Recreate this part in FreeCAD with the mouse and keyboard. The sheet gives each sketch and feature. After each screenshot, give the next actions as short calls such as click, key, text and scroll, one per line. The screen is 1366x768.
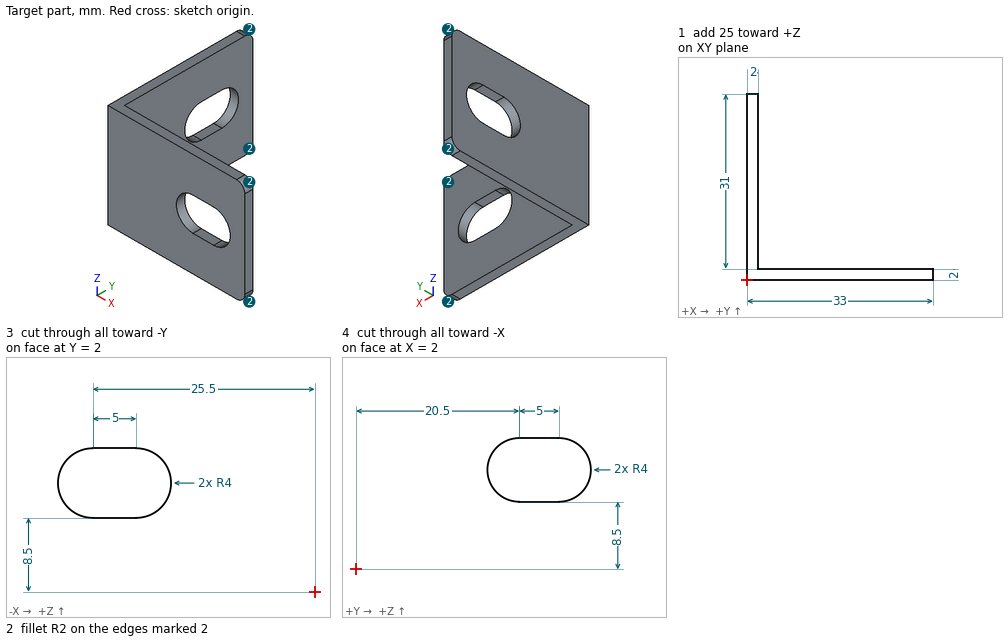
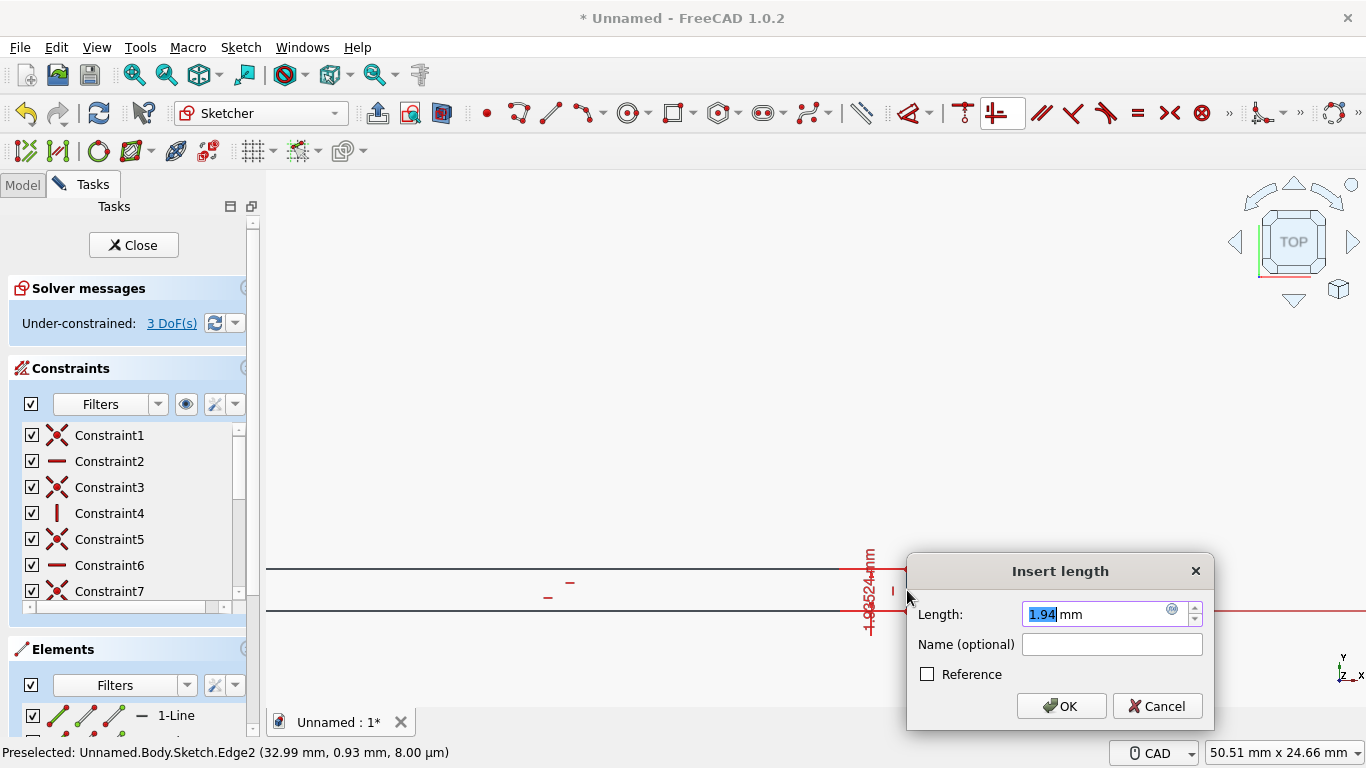
text(2)
key(Return)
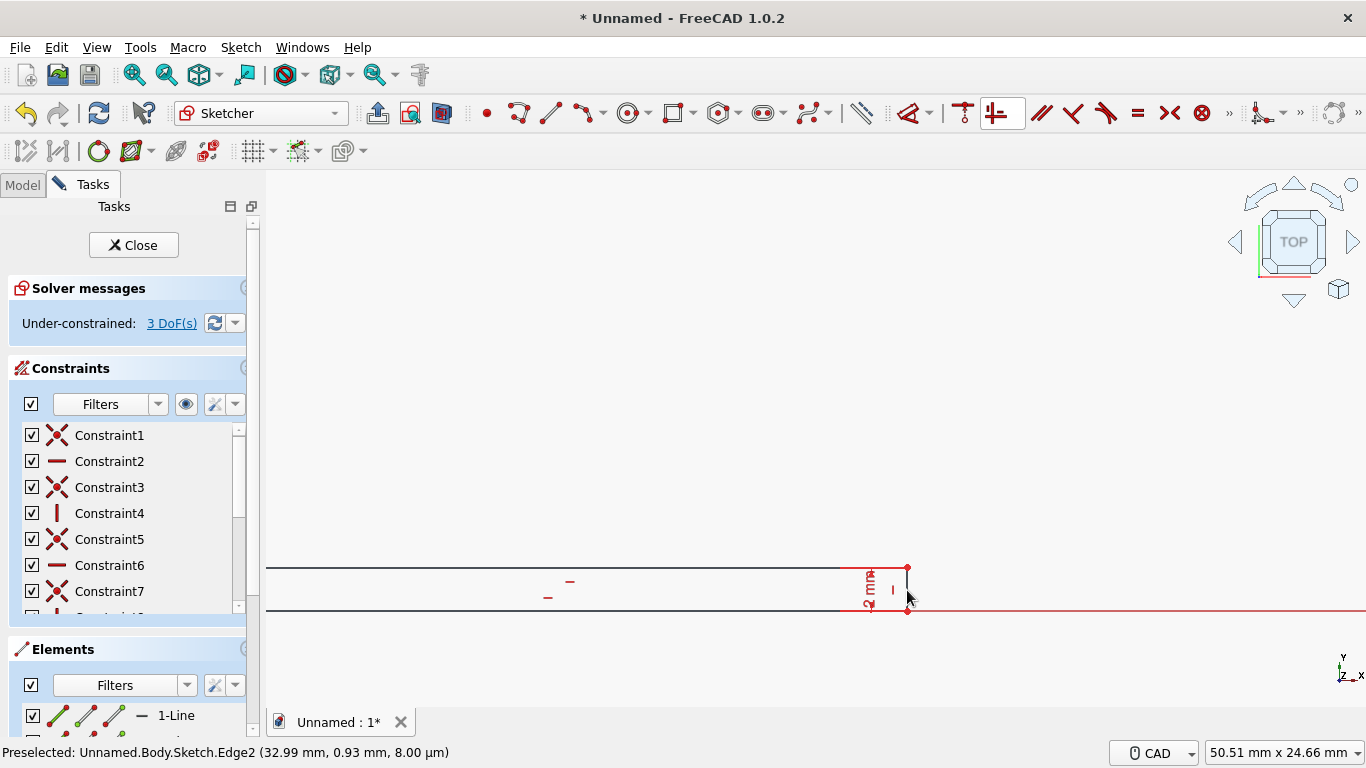
scroll(910, 591, down, 4)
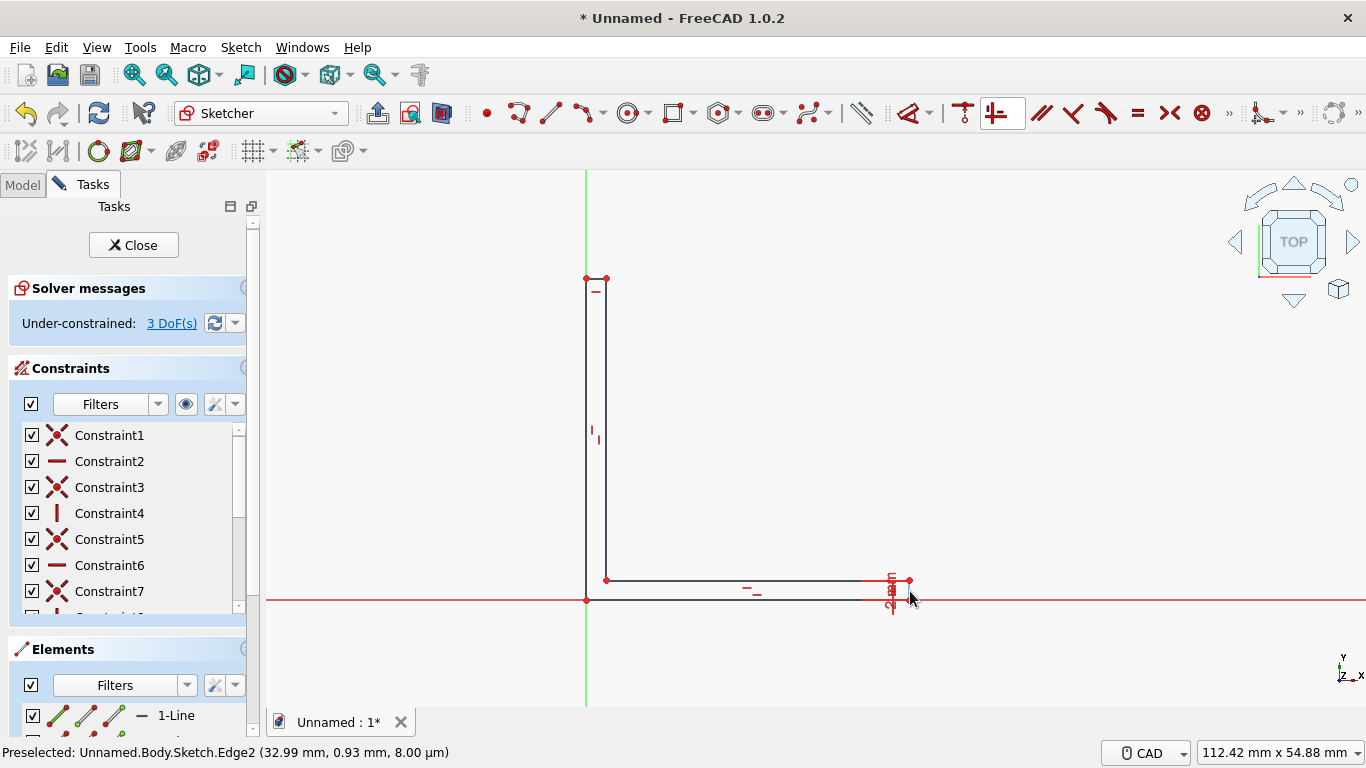
scroll(600, 279, up, 5)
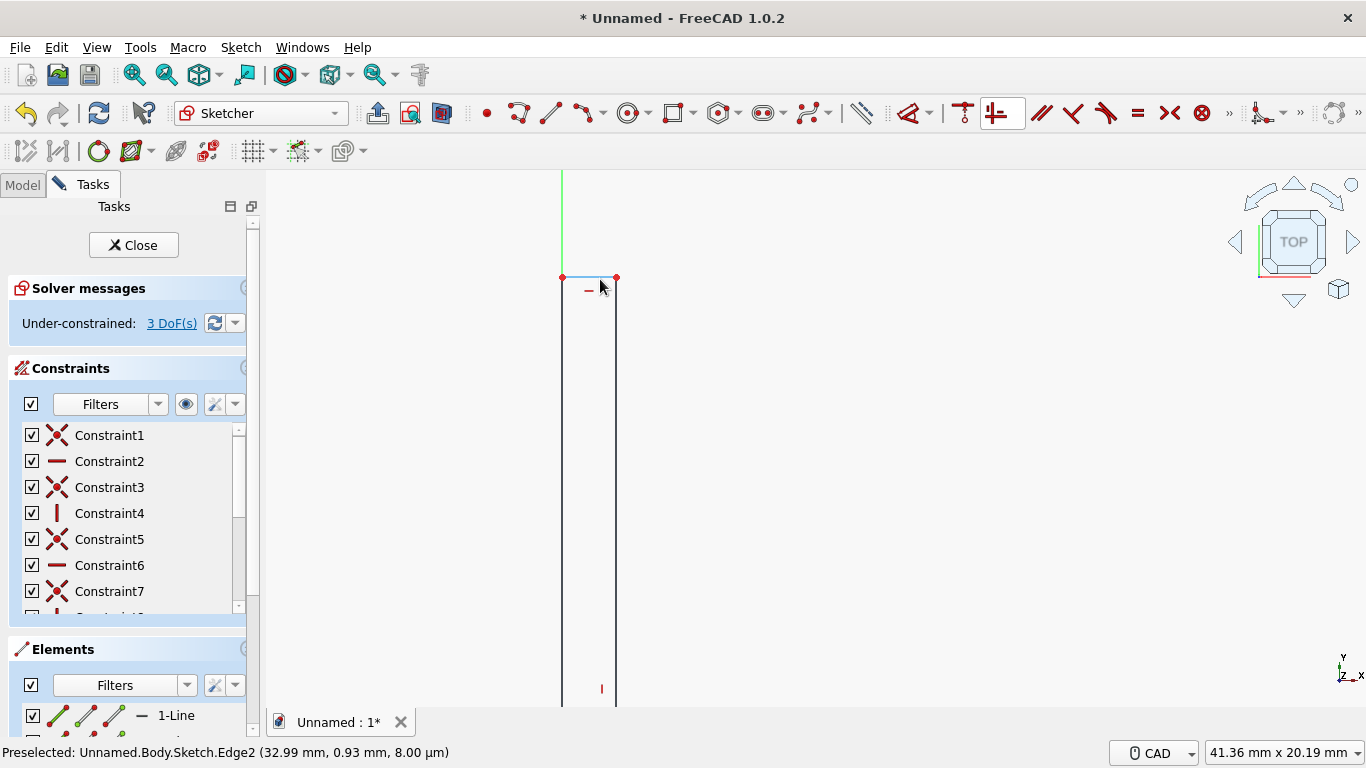
click(600, 277)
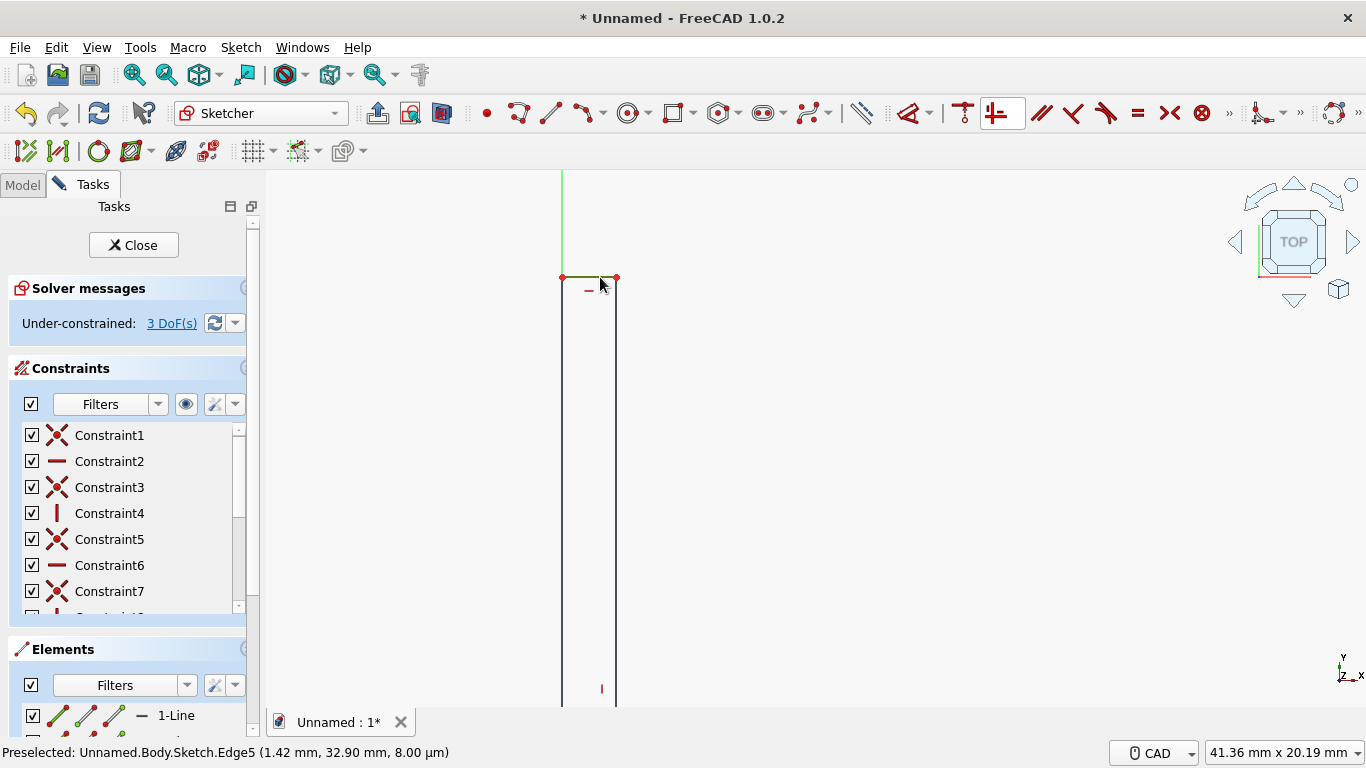
key(l)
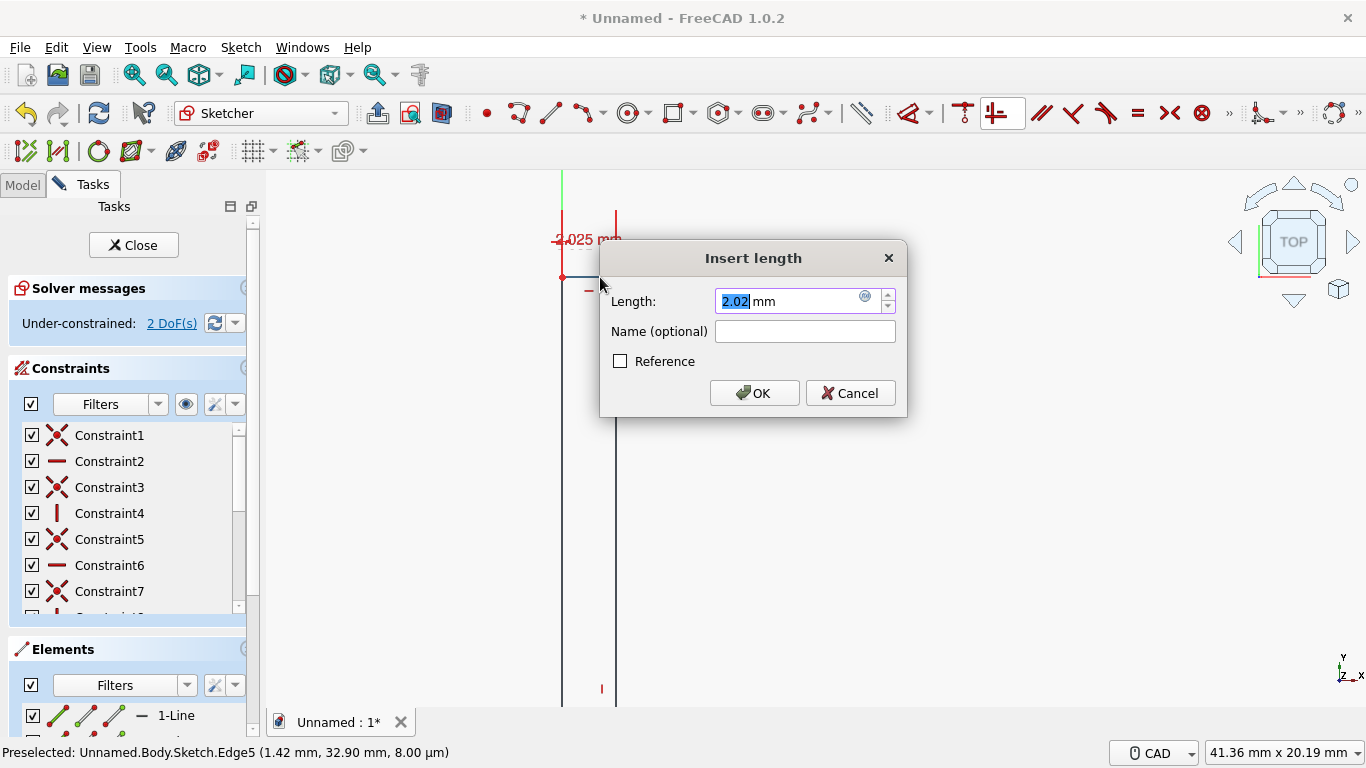
text(2)
key(Return)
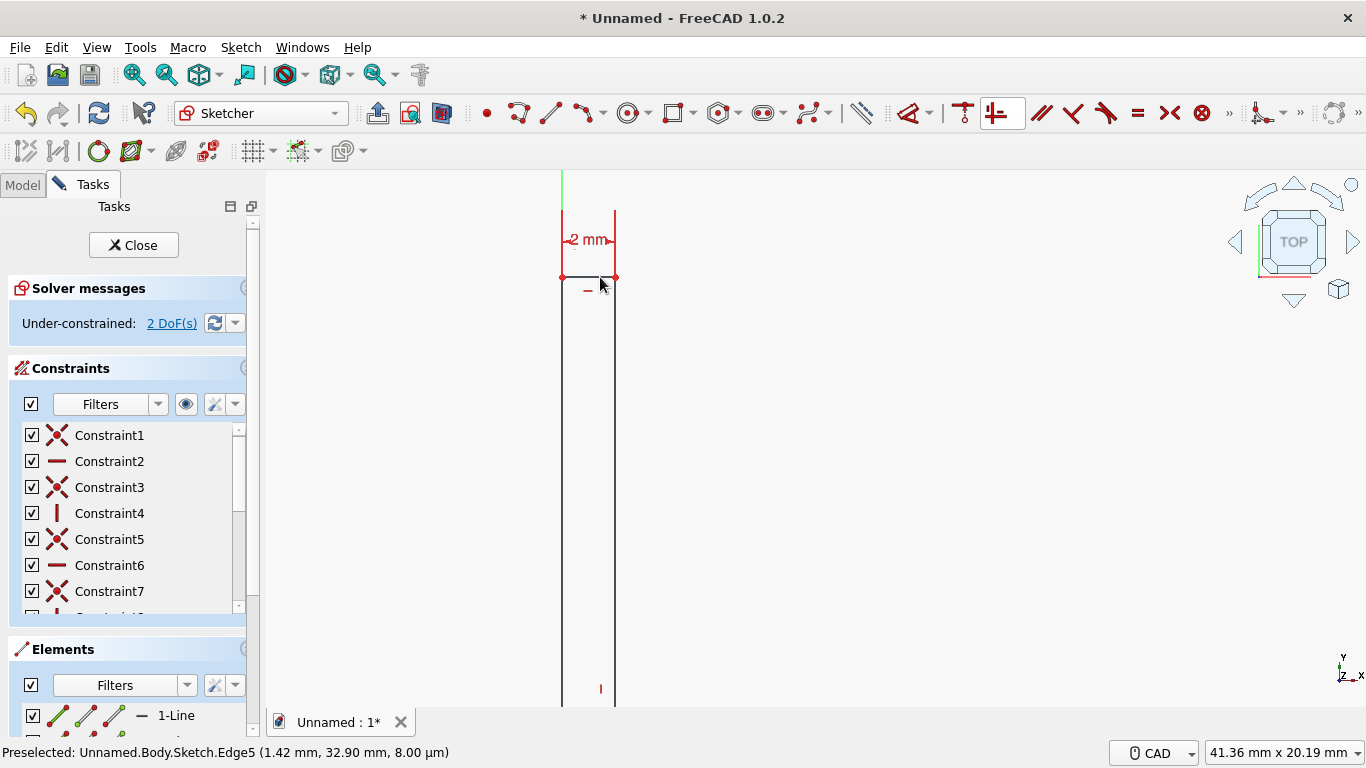
scroll(600, 278, down, 5)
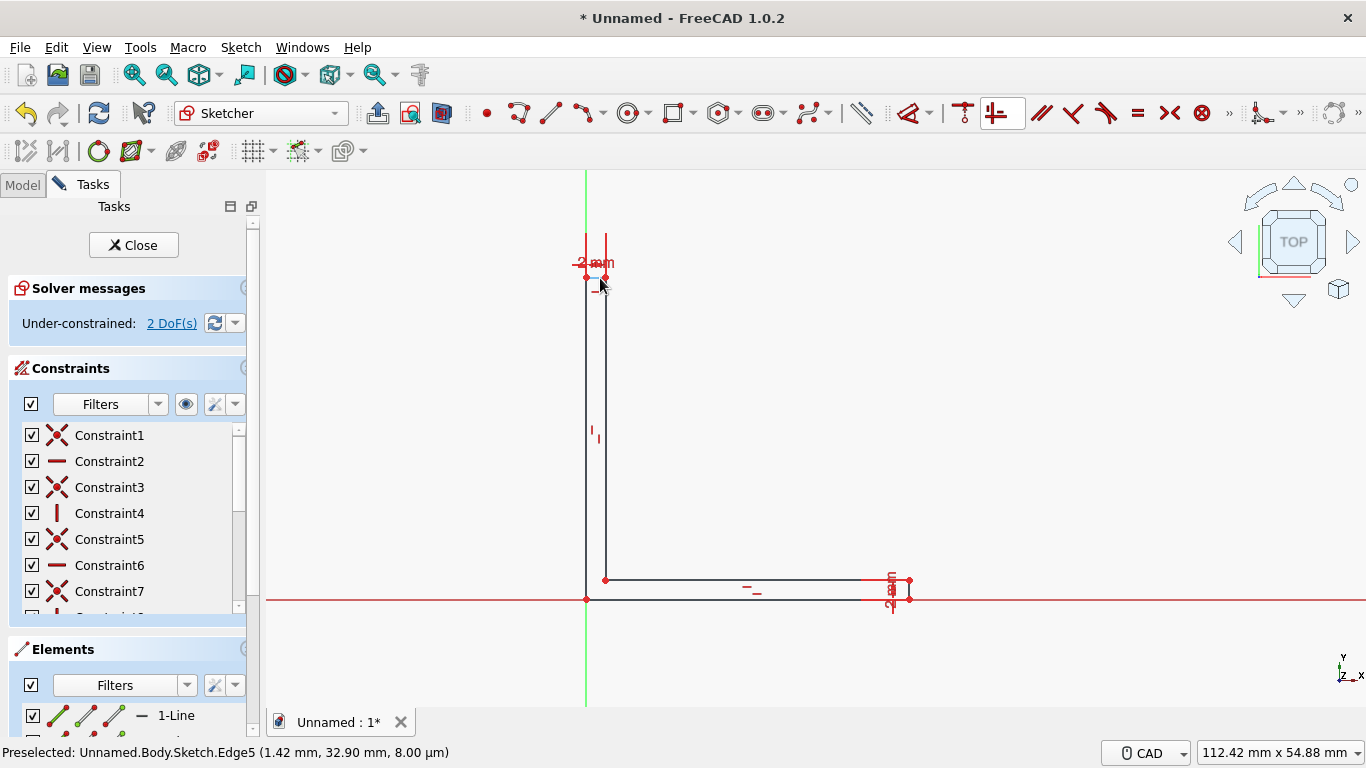
click(683, 600)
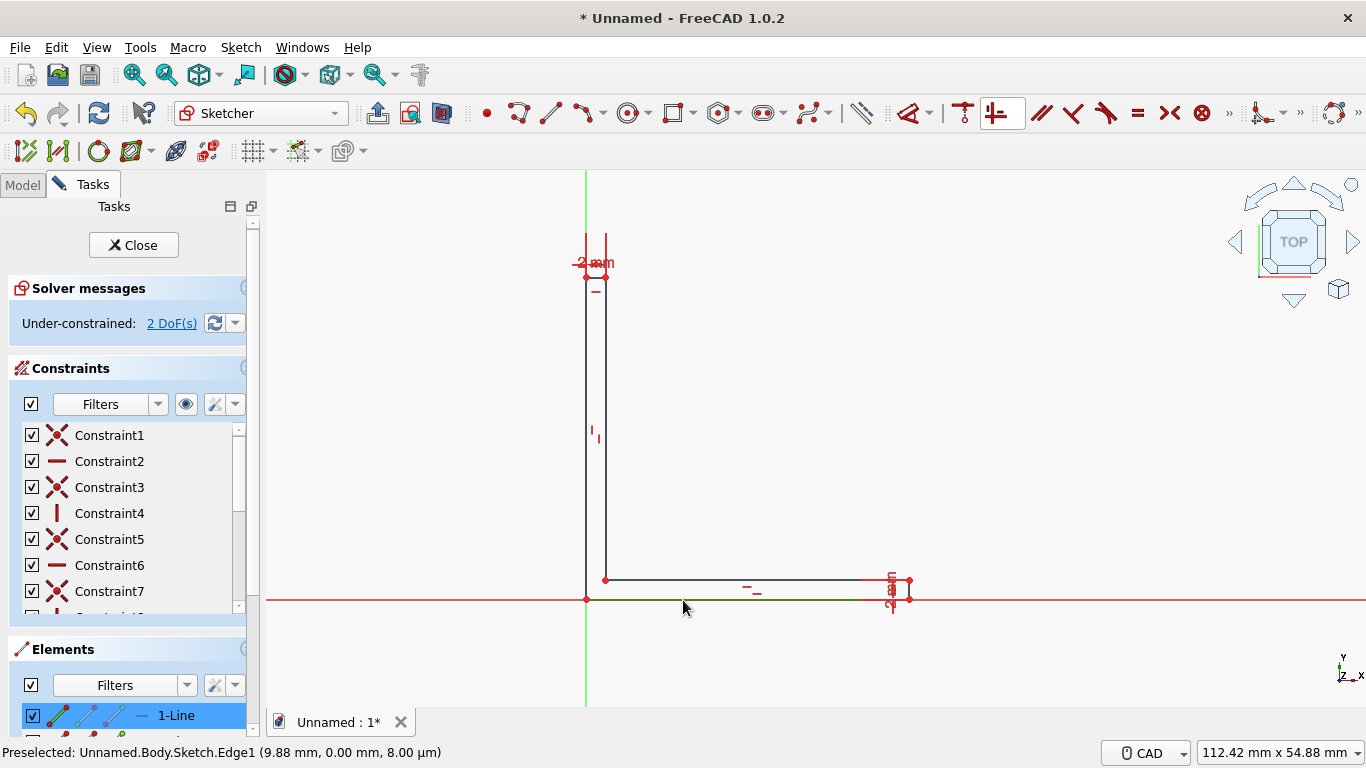
key(l)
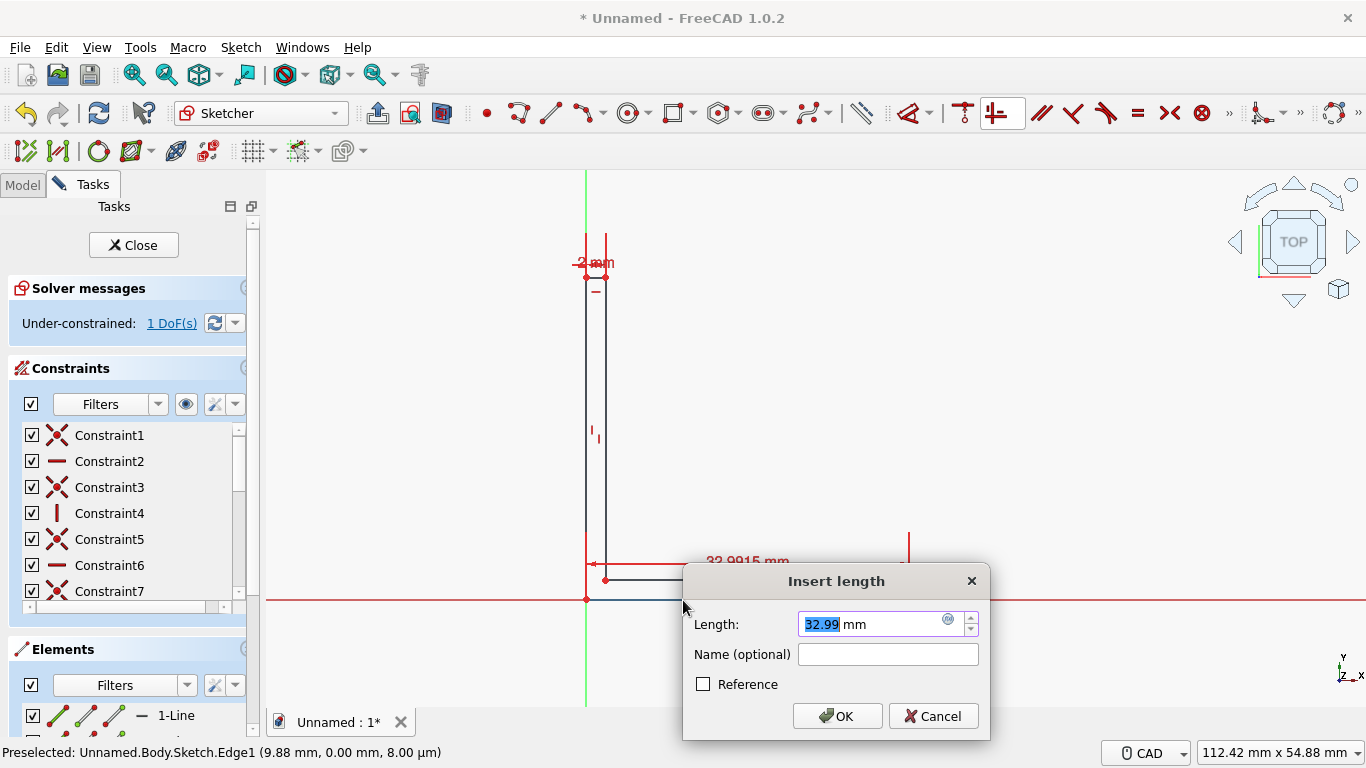
text(33)
key(Return)